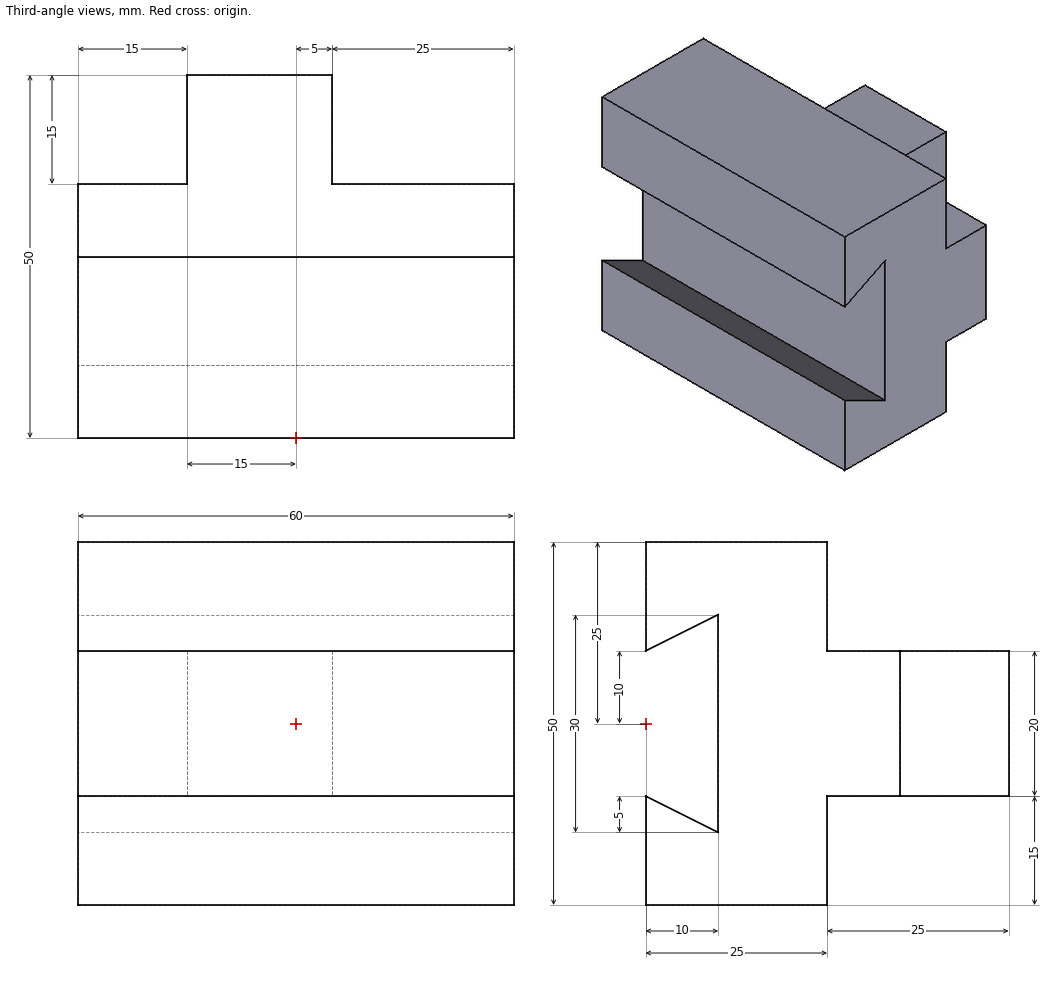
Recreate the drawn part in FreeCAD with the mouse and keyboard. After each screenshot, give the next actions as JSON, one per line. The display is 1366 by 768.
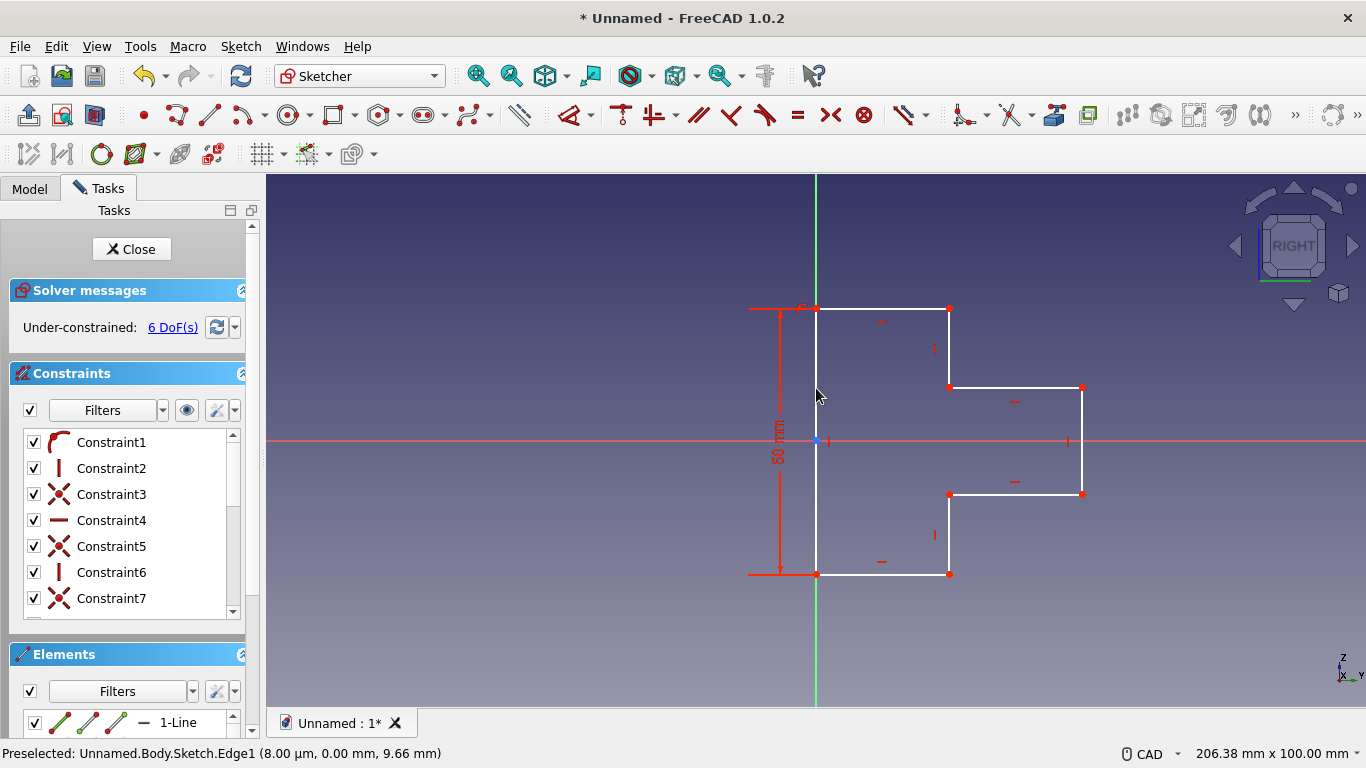
{"action": "left_click", "coordinate": [856, 575]}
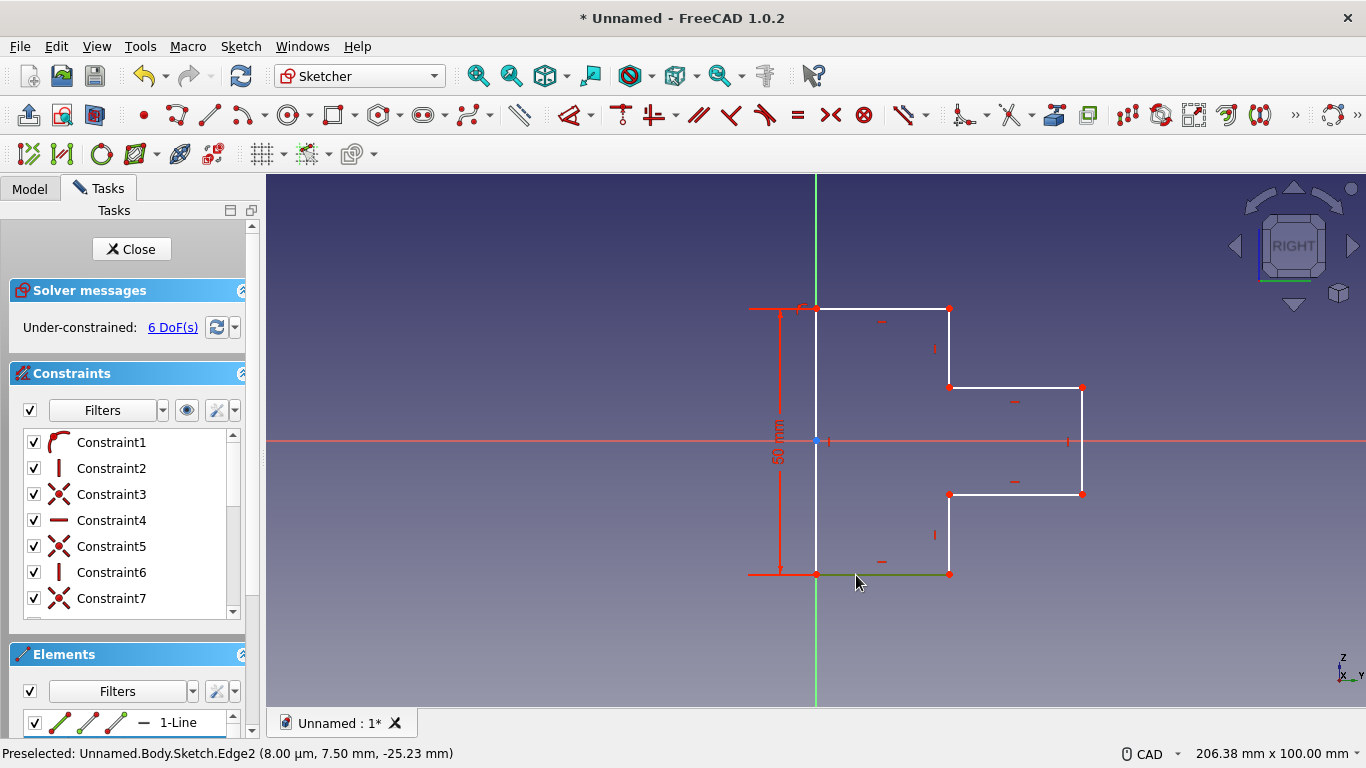
{"action": "left_click", "coordinate": [590, 116]}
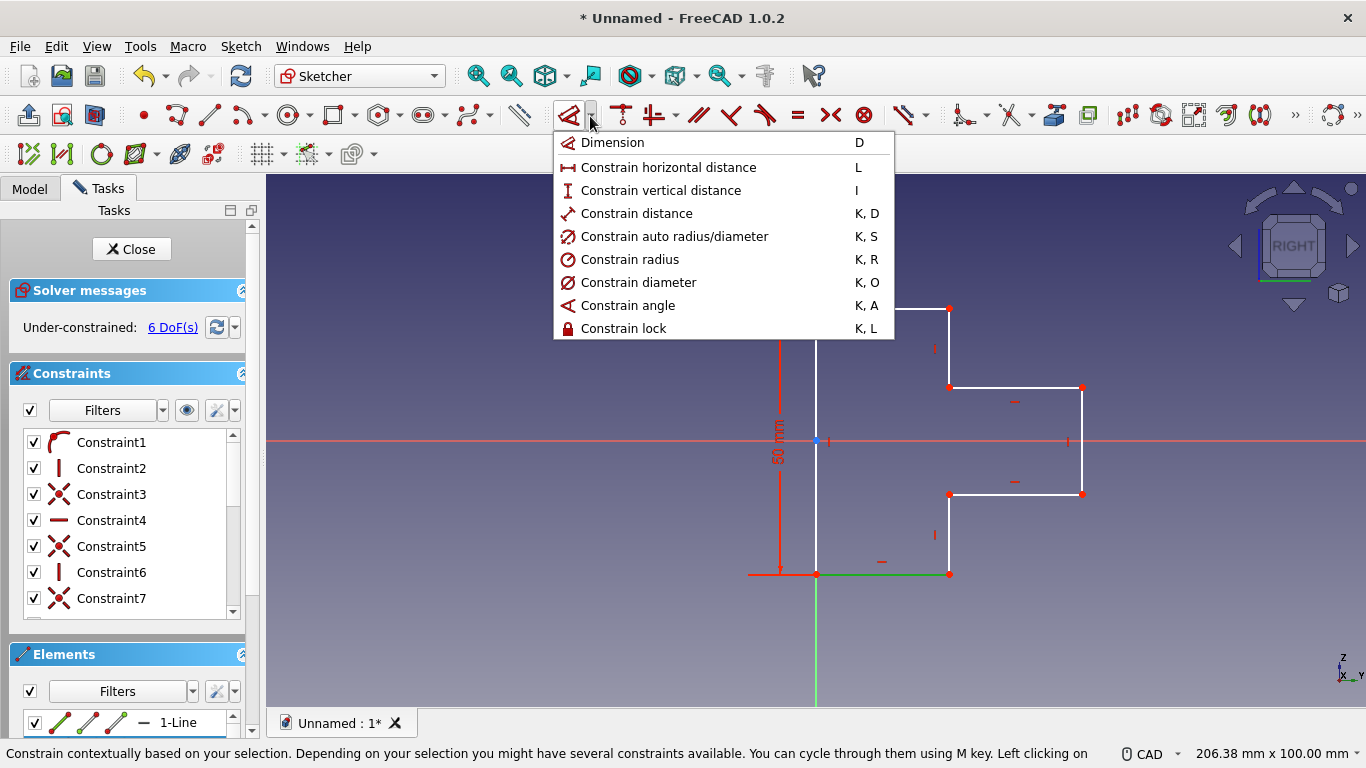
{"action": "left_click", "coordinate": [724, 168]}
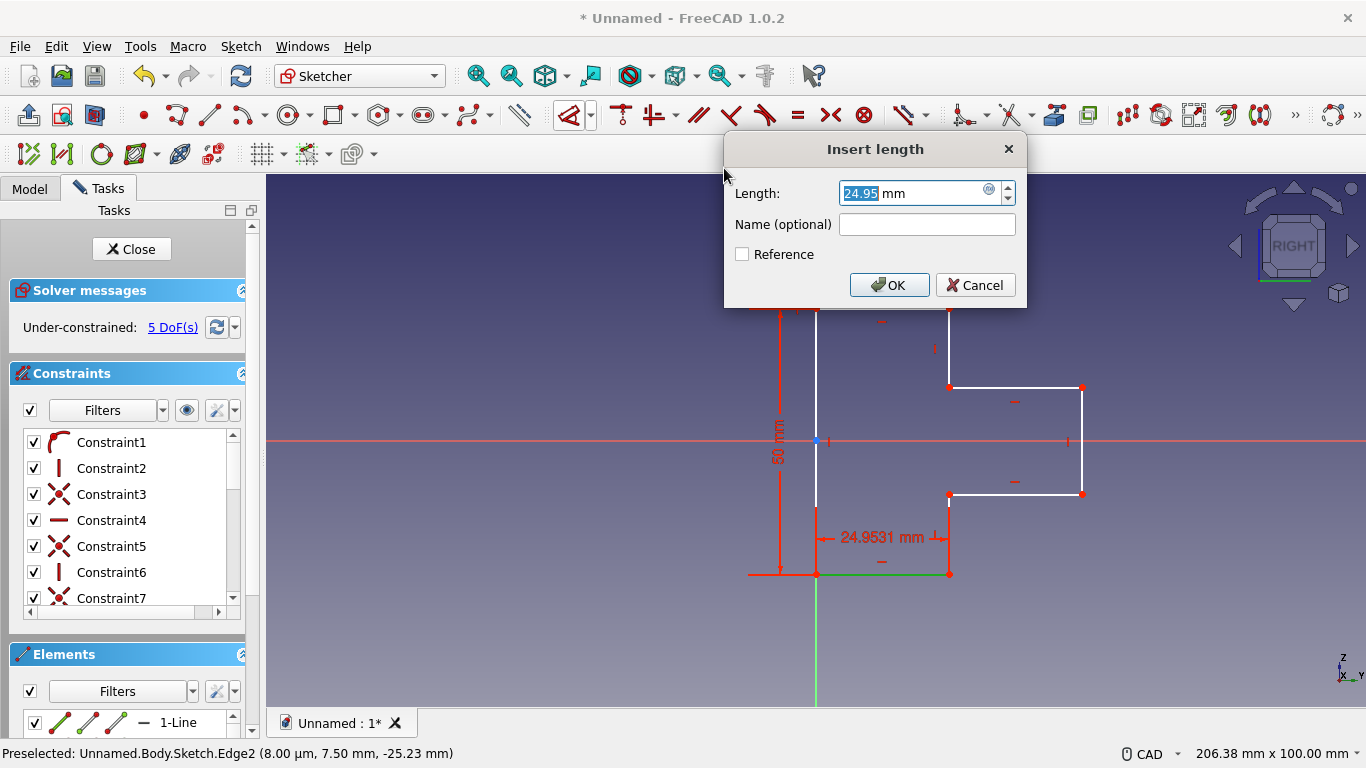
{"action": "type", "text": "25"}
{"action": "key", "text": "Return"}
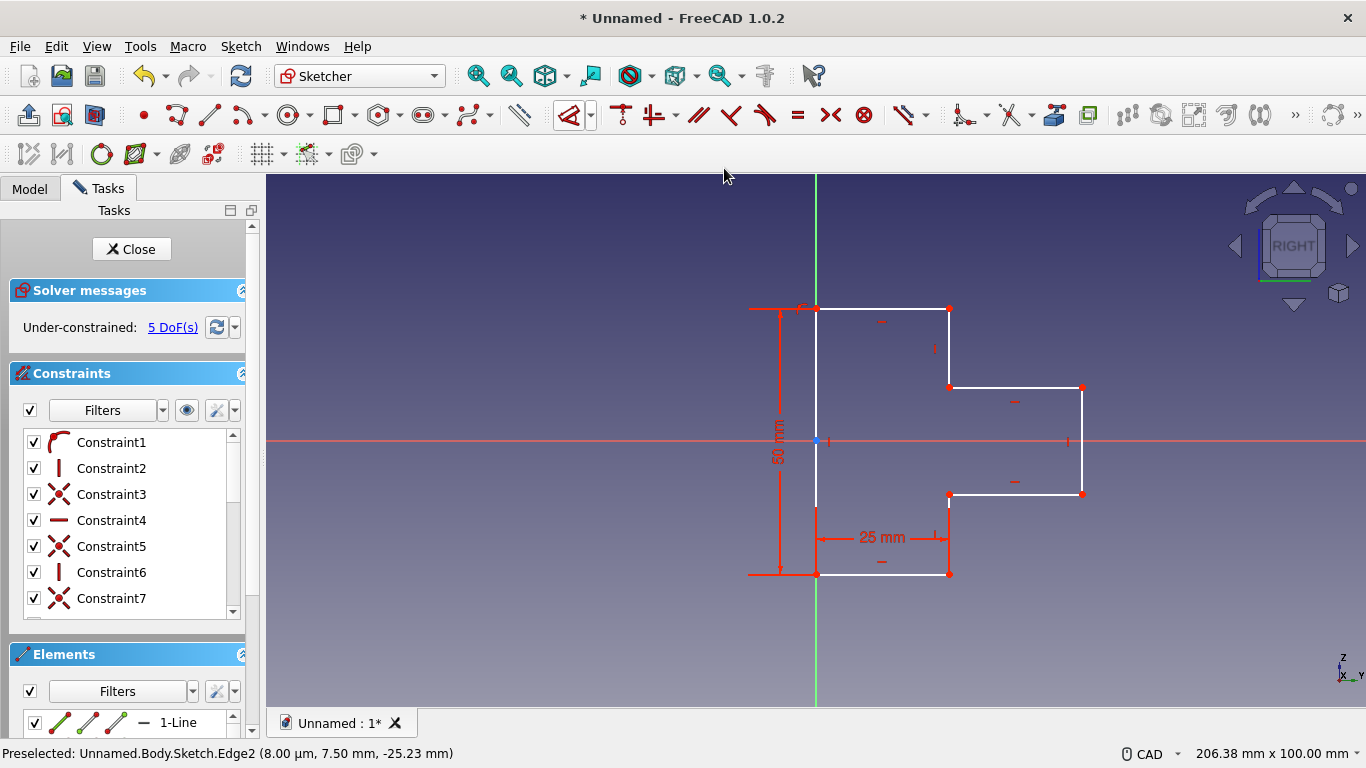
{"action": "left_click", "coordinate": [949, 551]}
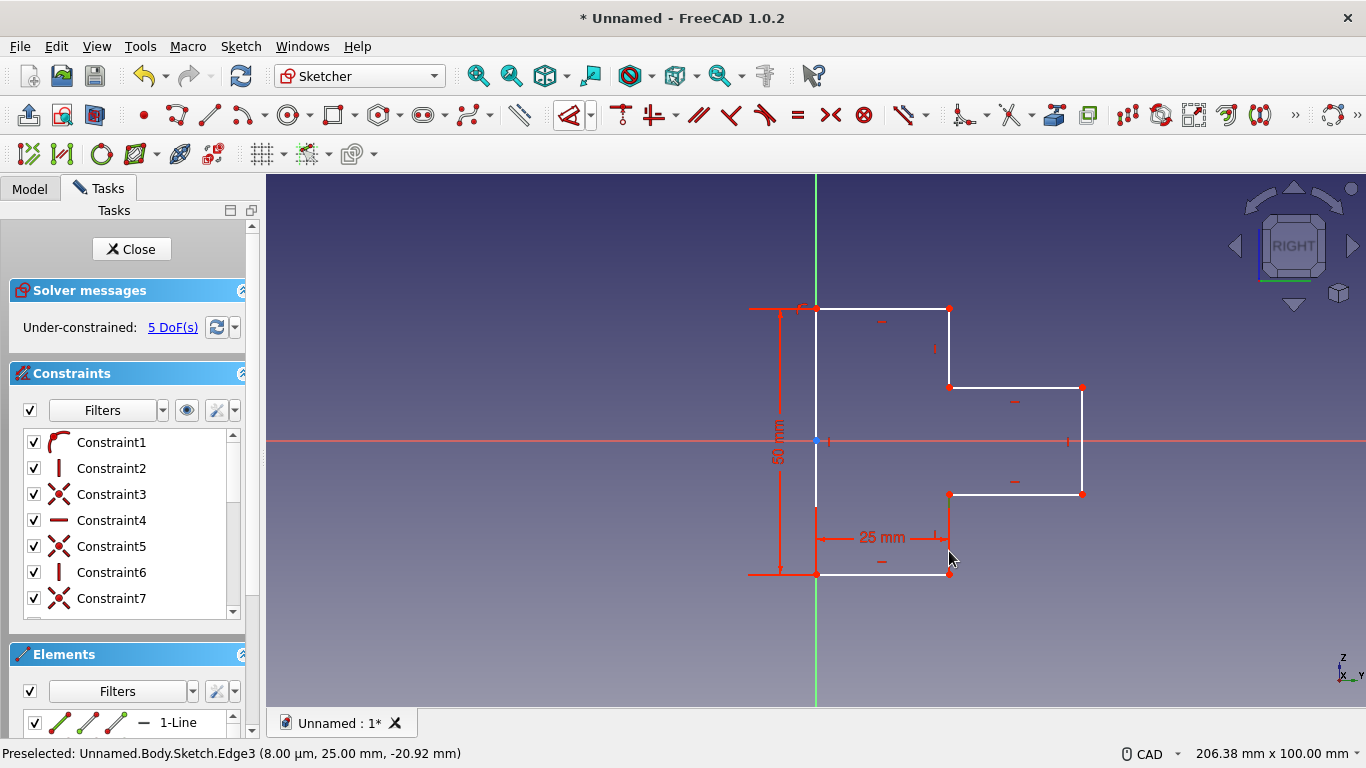
{"action": "left_click", "coordinate": [590, 116]}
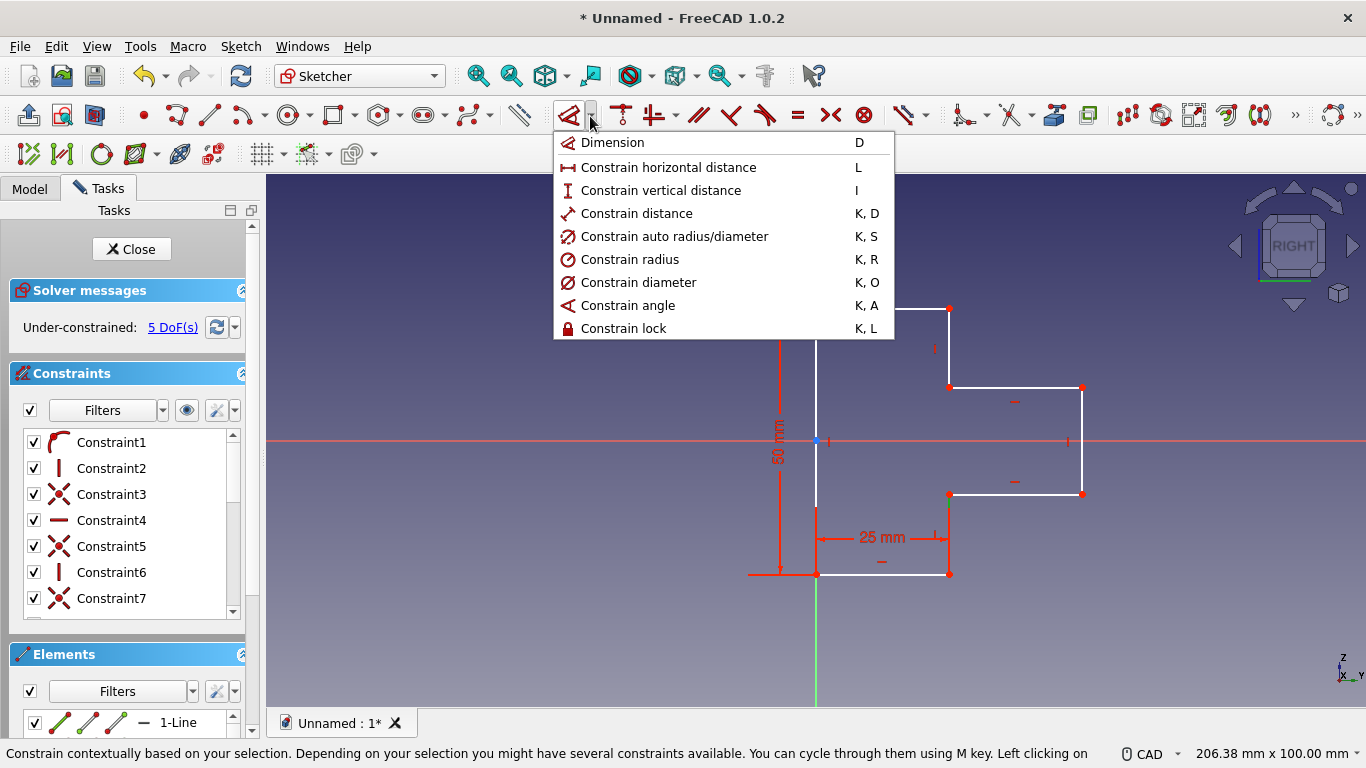
{"action": "left_click", "coordinate": [724, 190]}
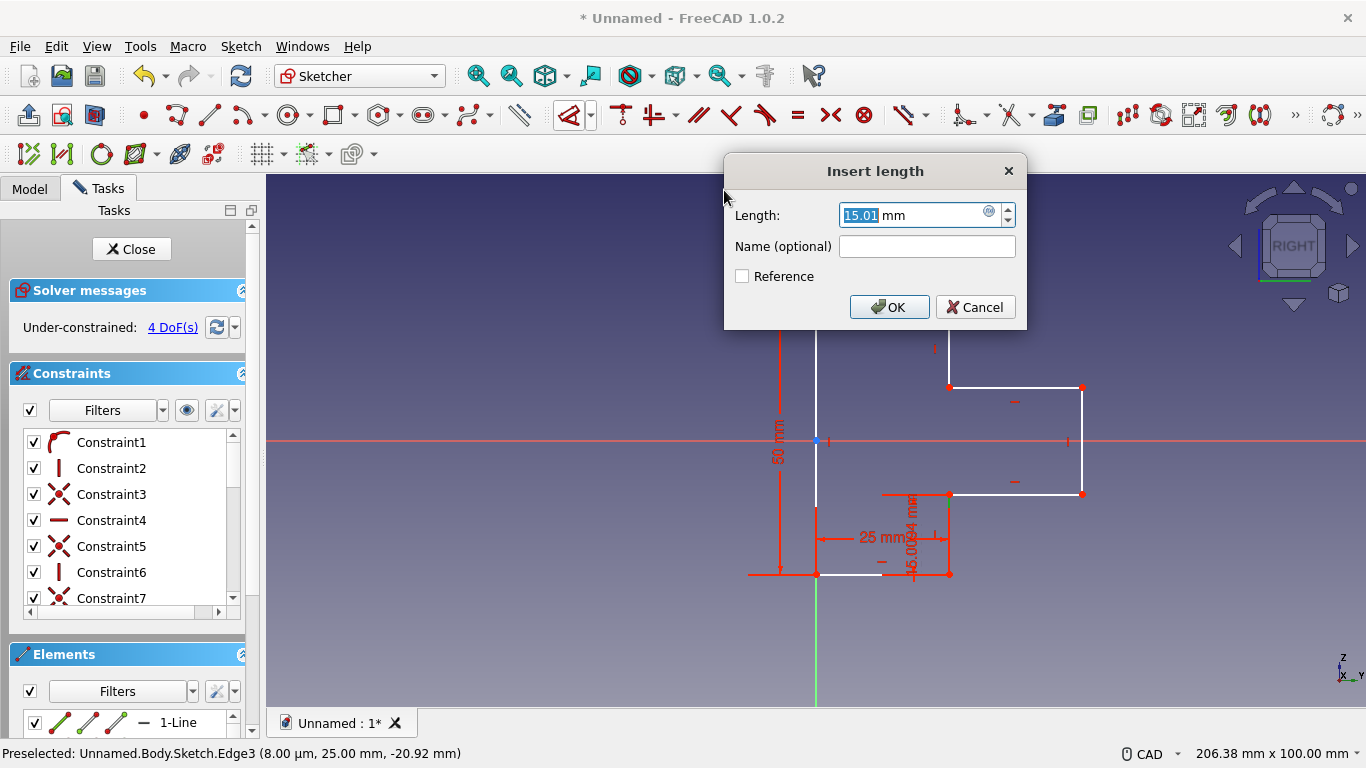
{"action": "type", "text": "15"}
{"action": "key", "text": "Return"}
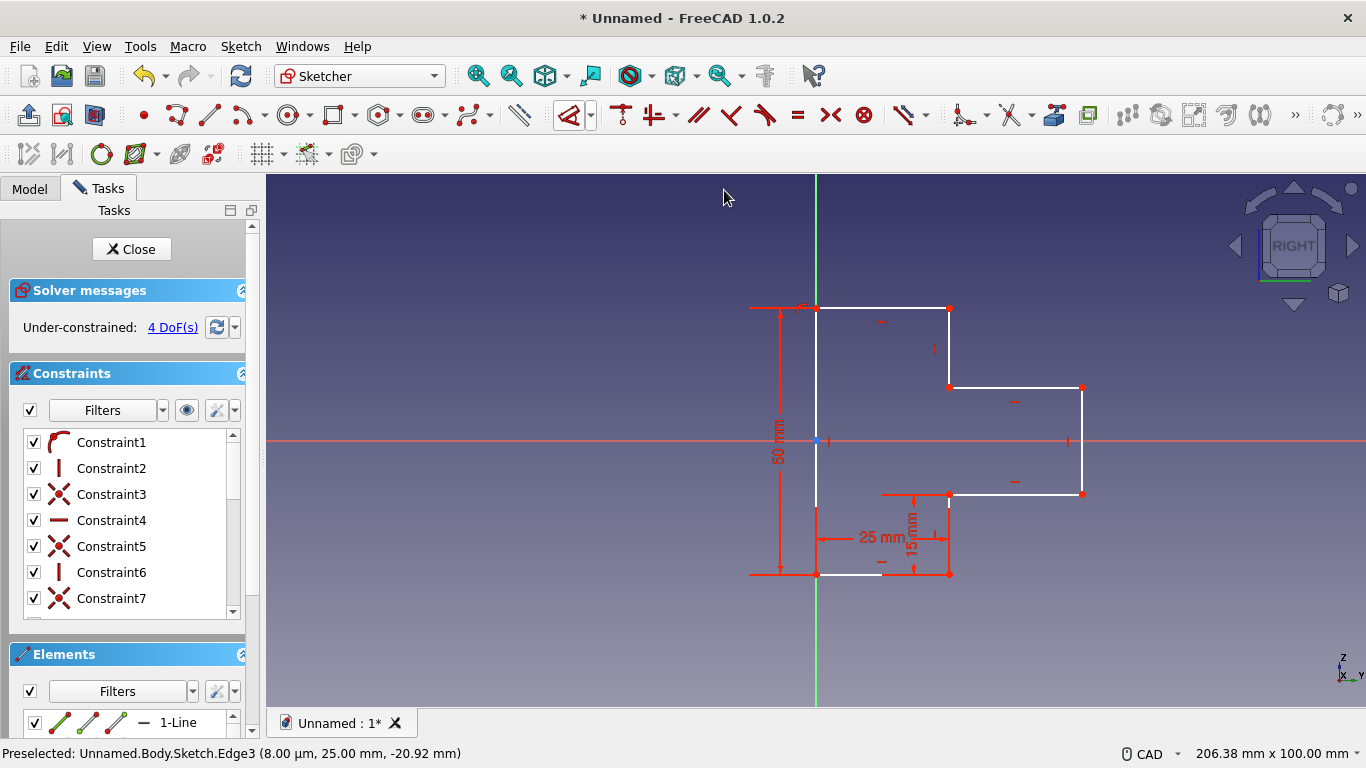
{"action": "left_click", "coordinate": [989, 495]}